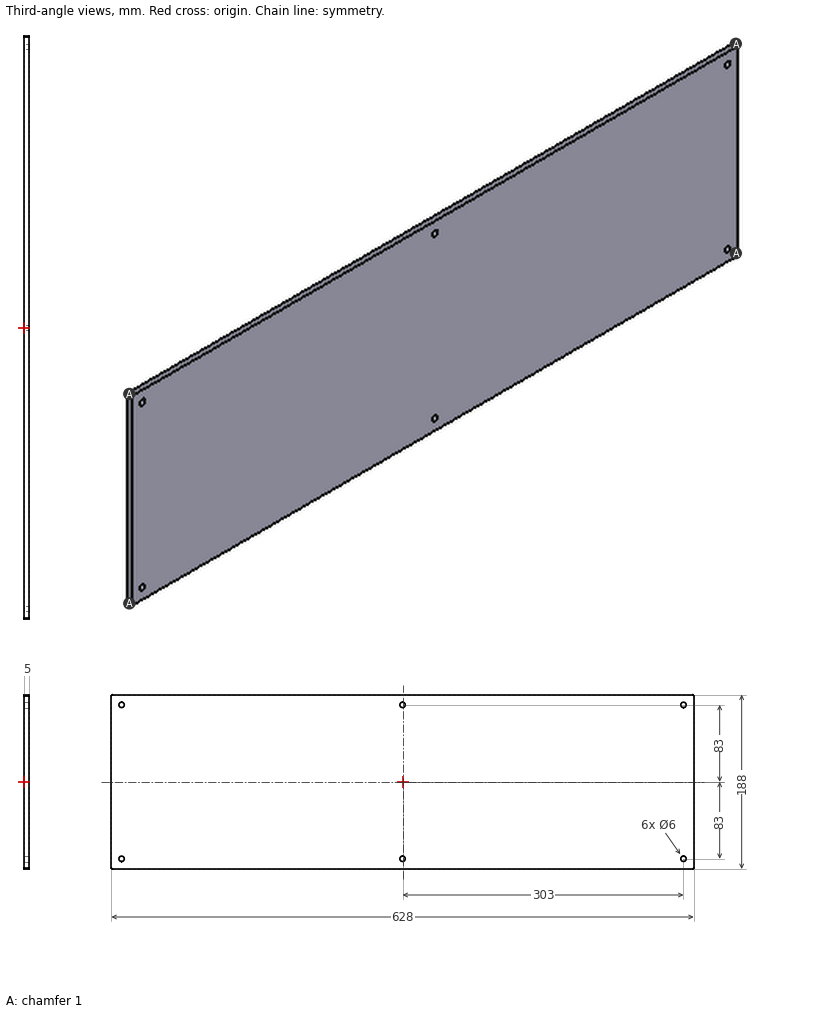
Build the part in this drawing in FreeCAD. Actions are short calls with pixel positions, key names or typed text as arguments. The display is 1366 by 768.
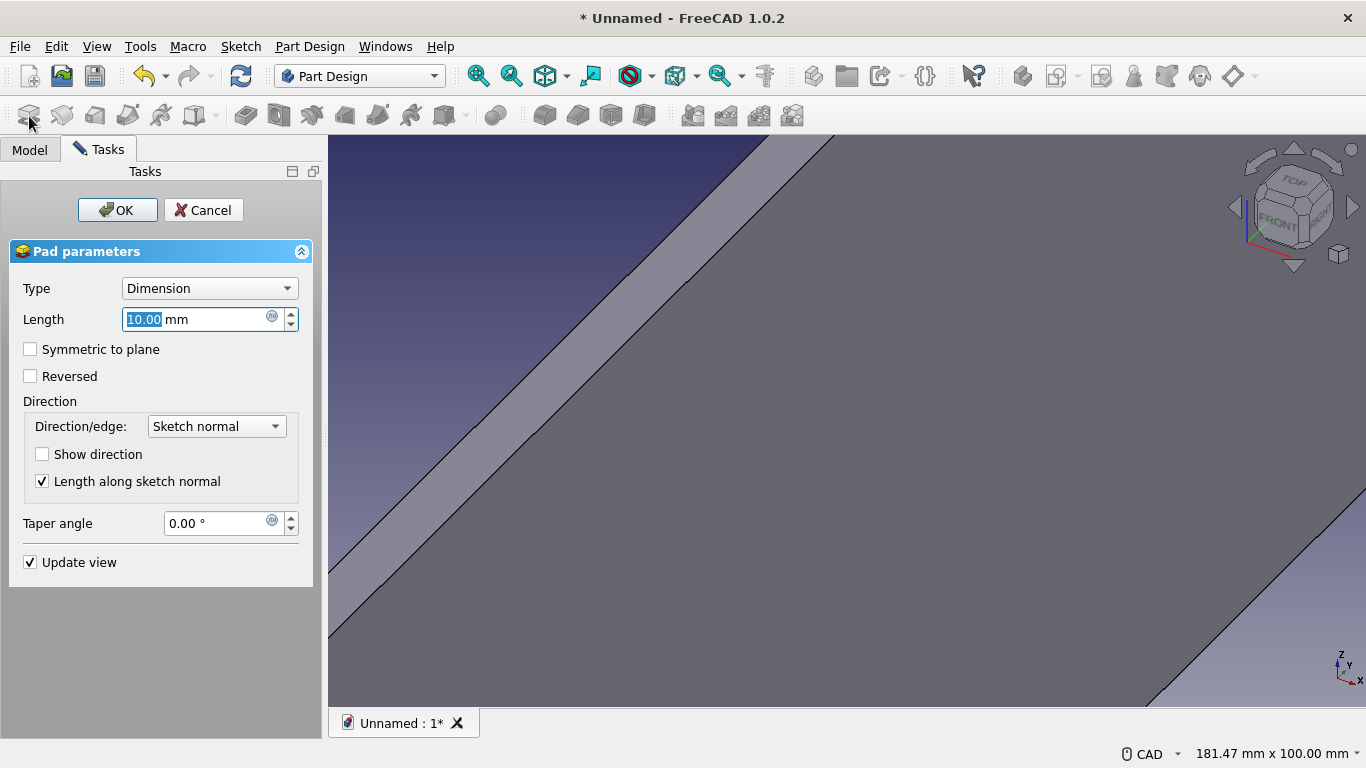
text(5)
key(Tab)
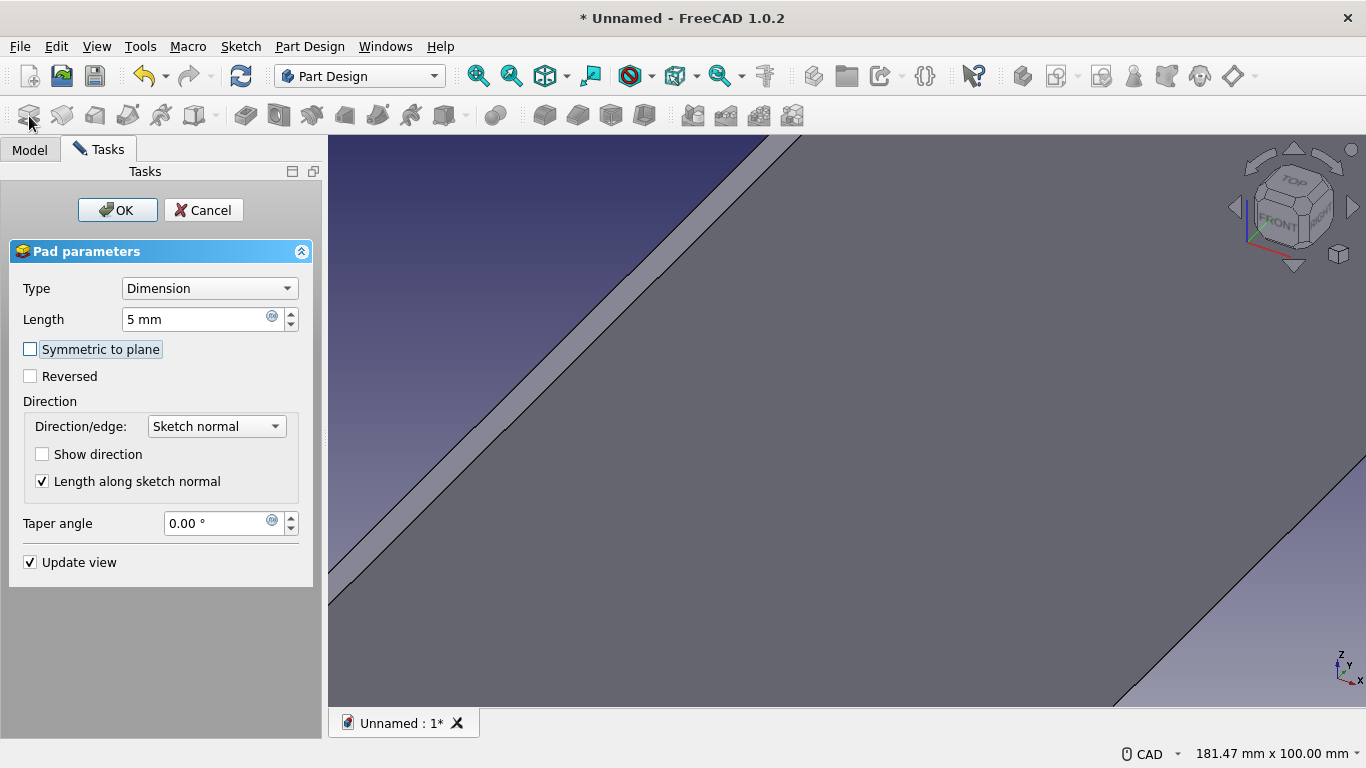
click(118, 210)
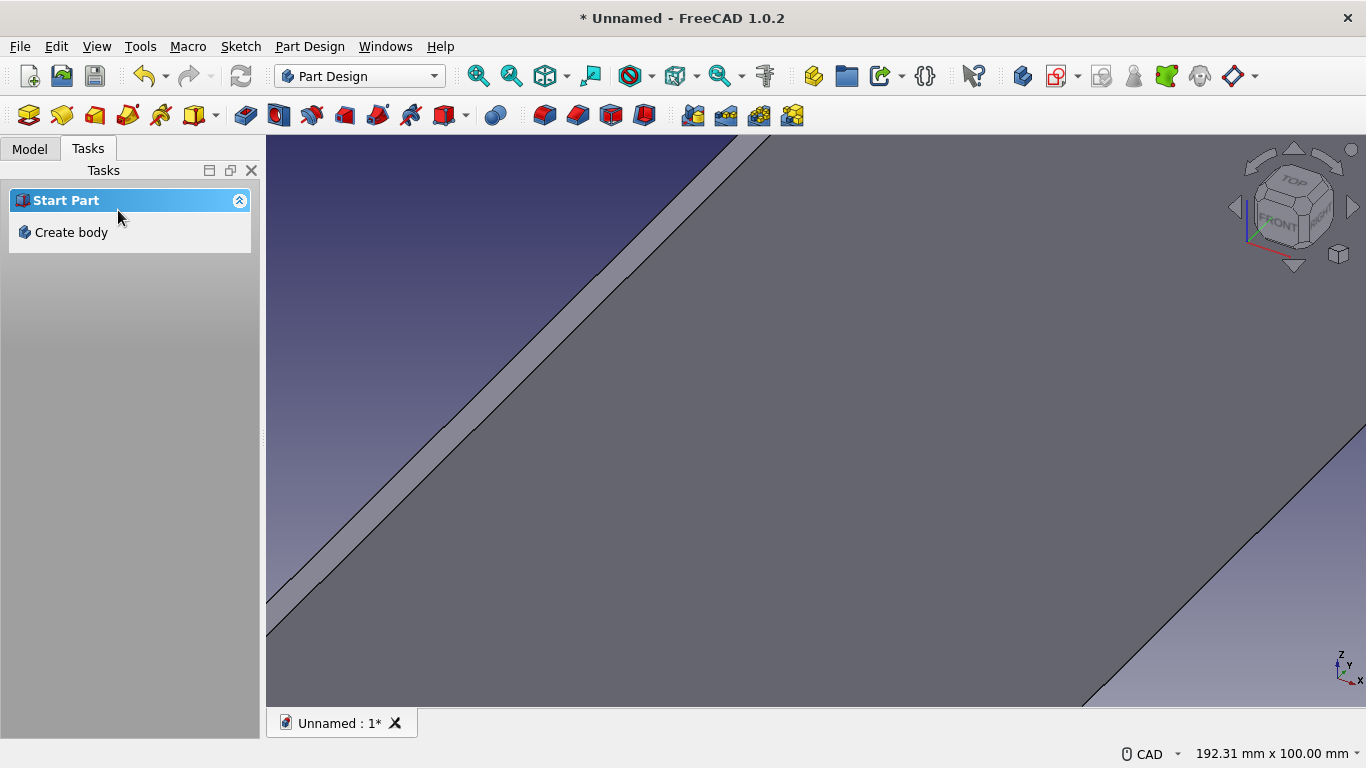
click(479, 76)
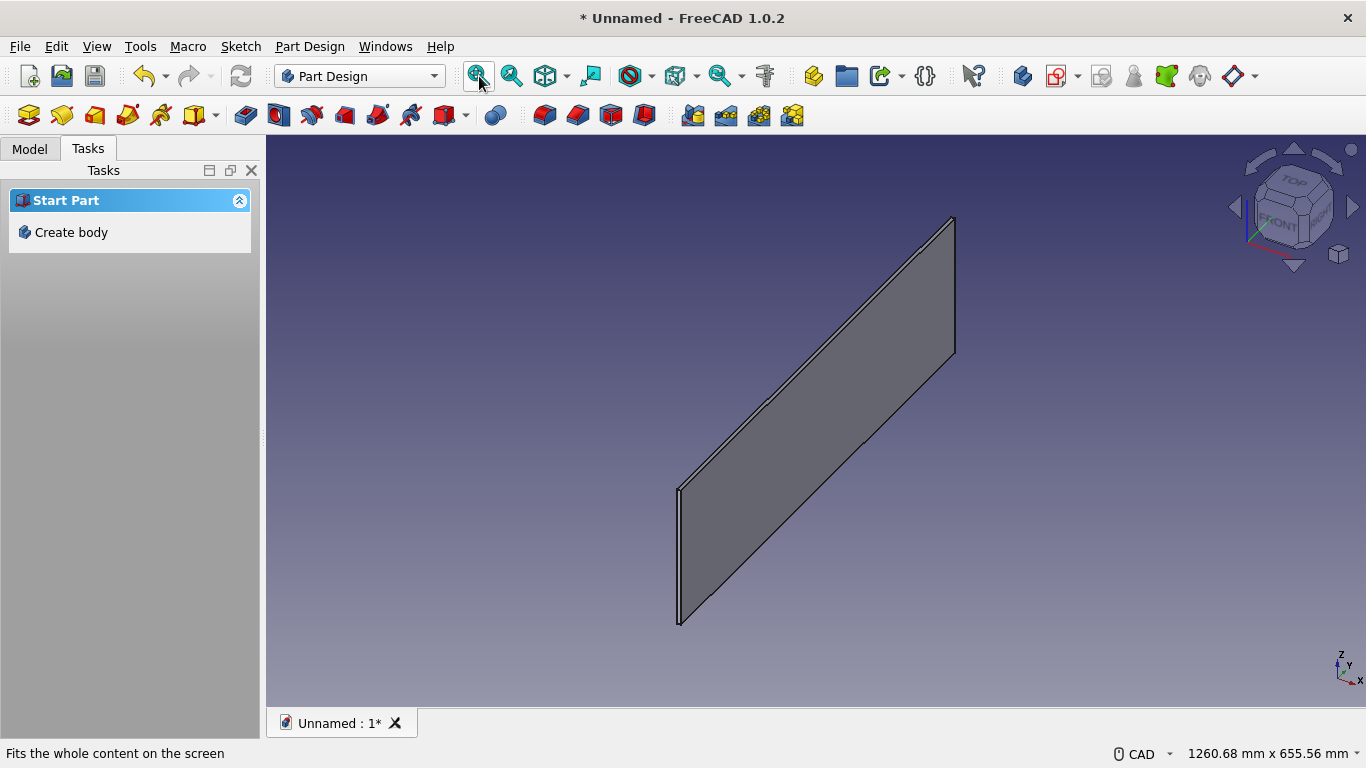
scroll(953, 217, up, 12)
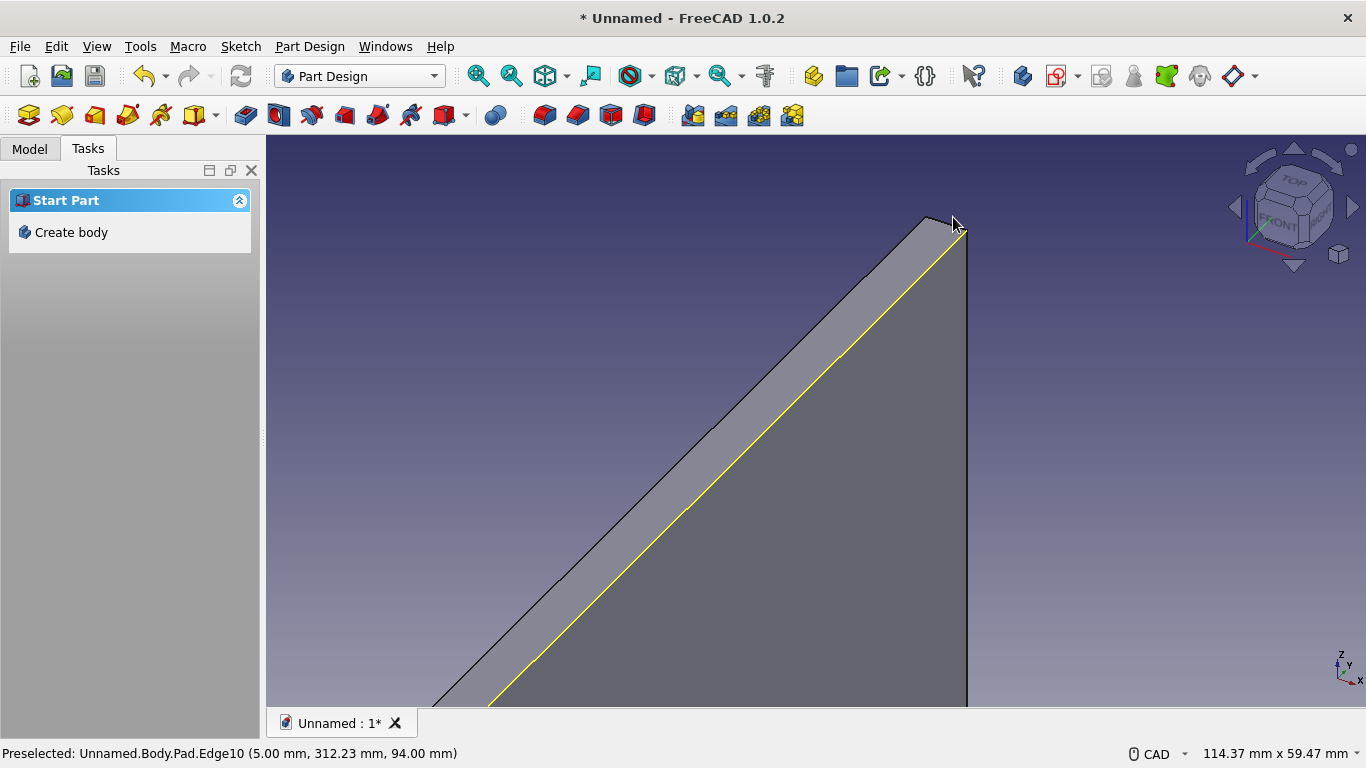
click(479, 76)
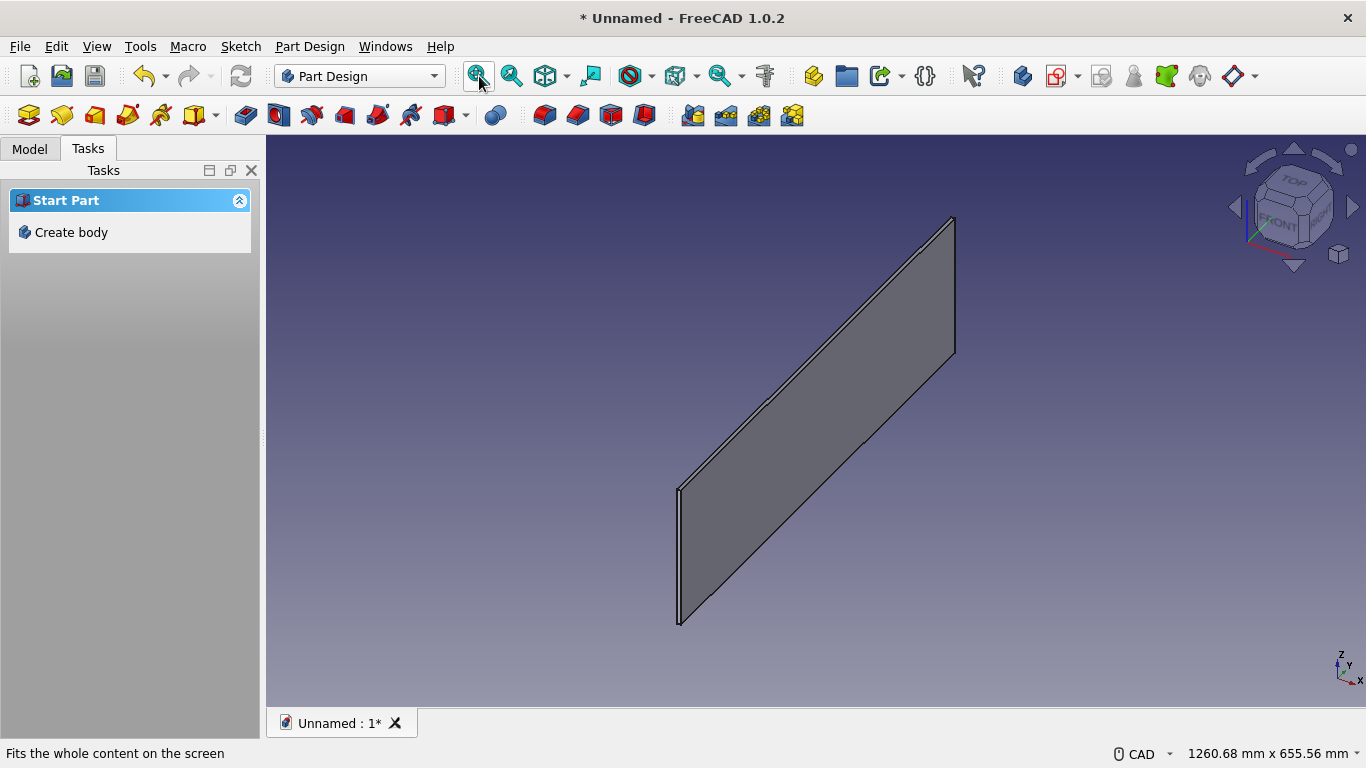
key(0)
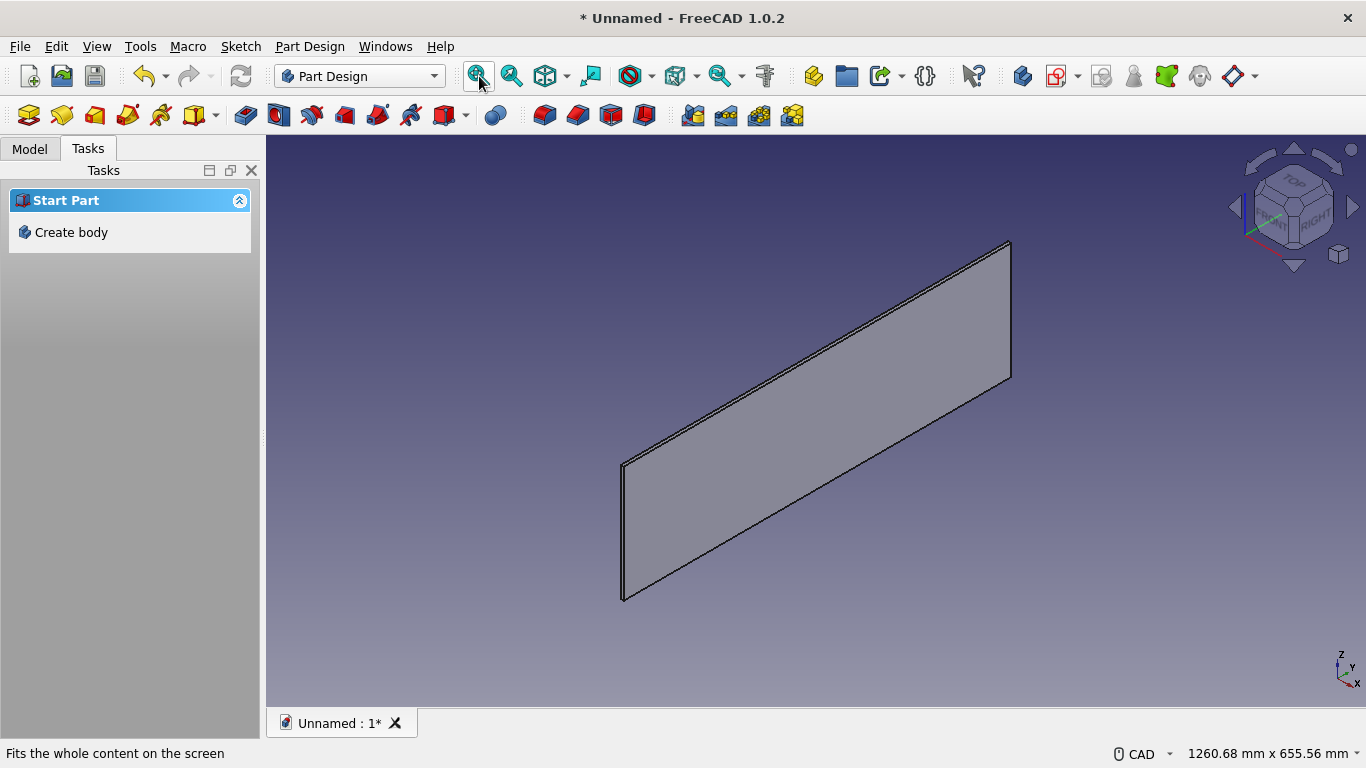
scroll(1010, 241, up, 12)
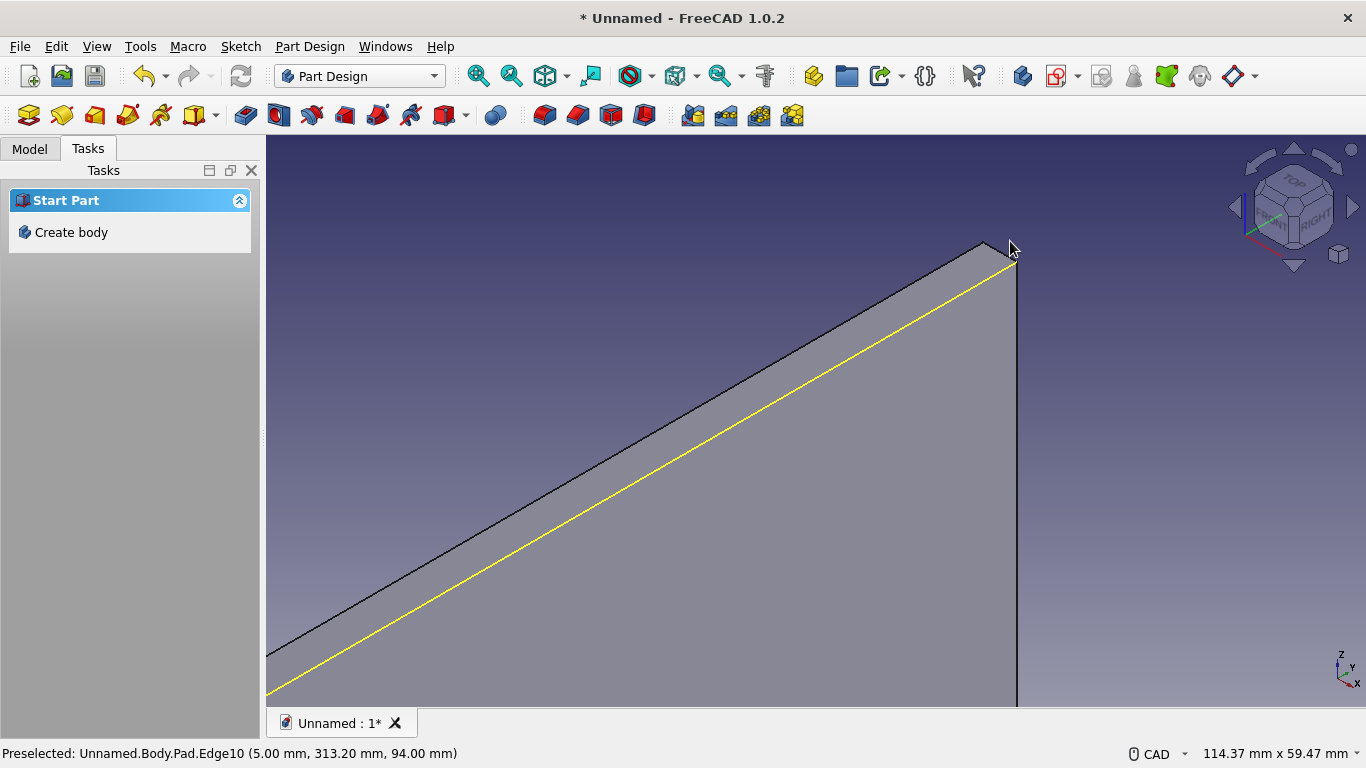
key(v)
key(f)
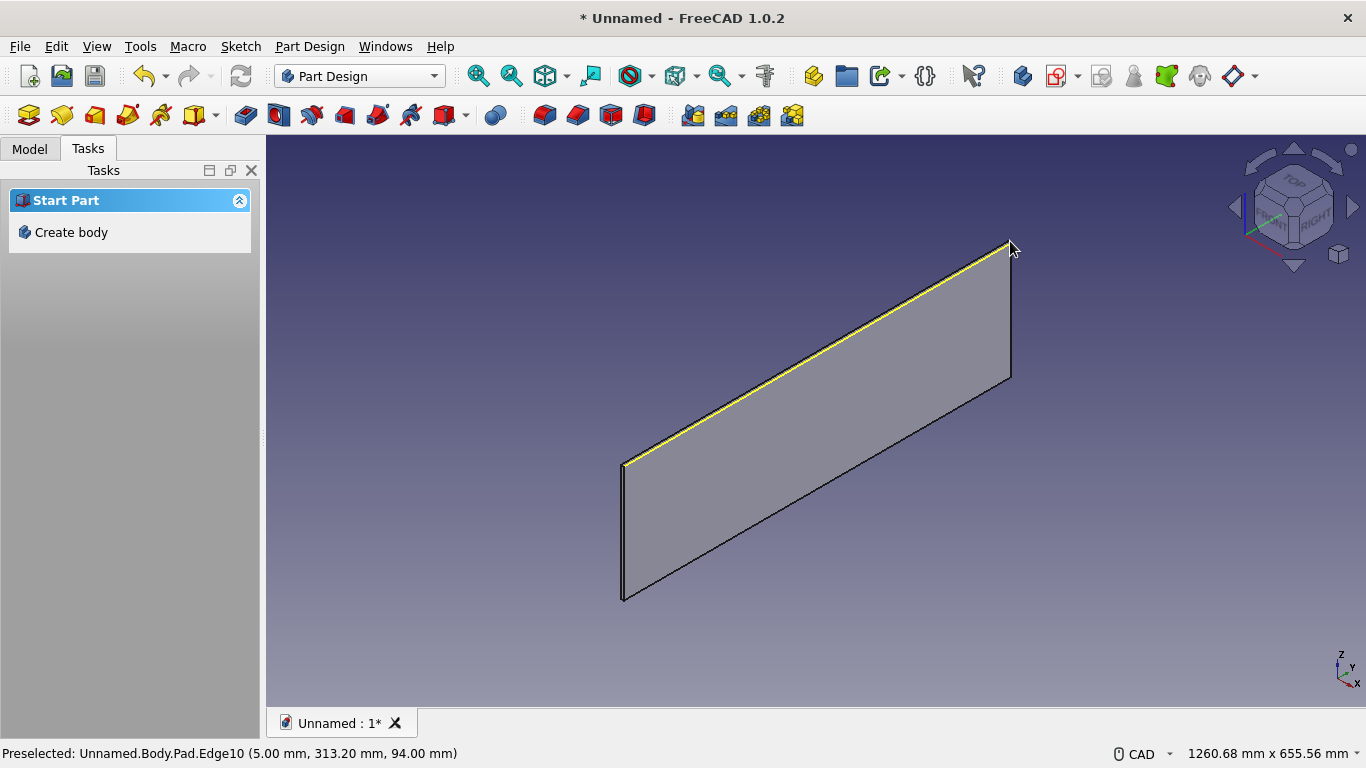
key(2)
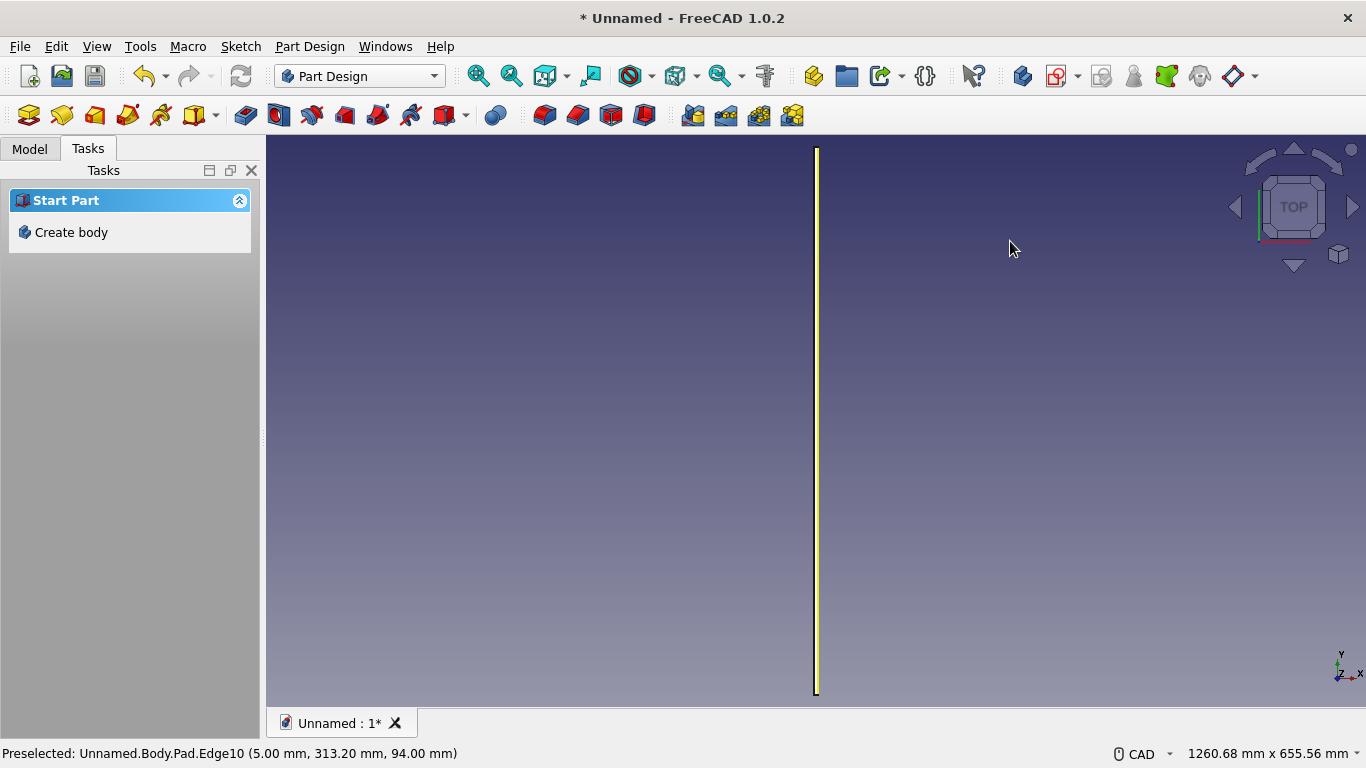
key(1)